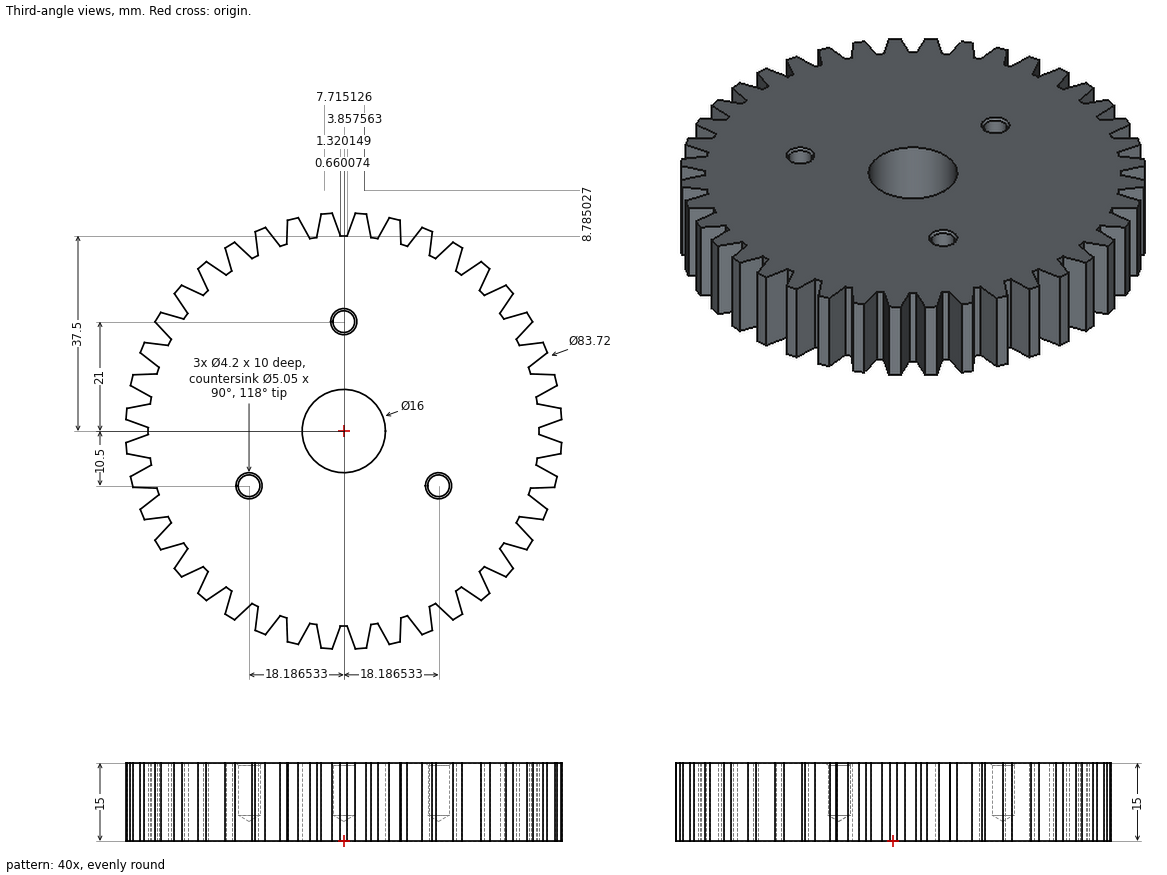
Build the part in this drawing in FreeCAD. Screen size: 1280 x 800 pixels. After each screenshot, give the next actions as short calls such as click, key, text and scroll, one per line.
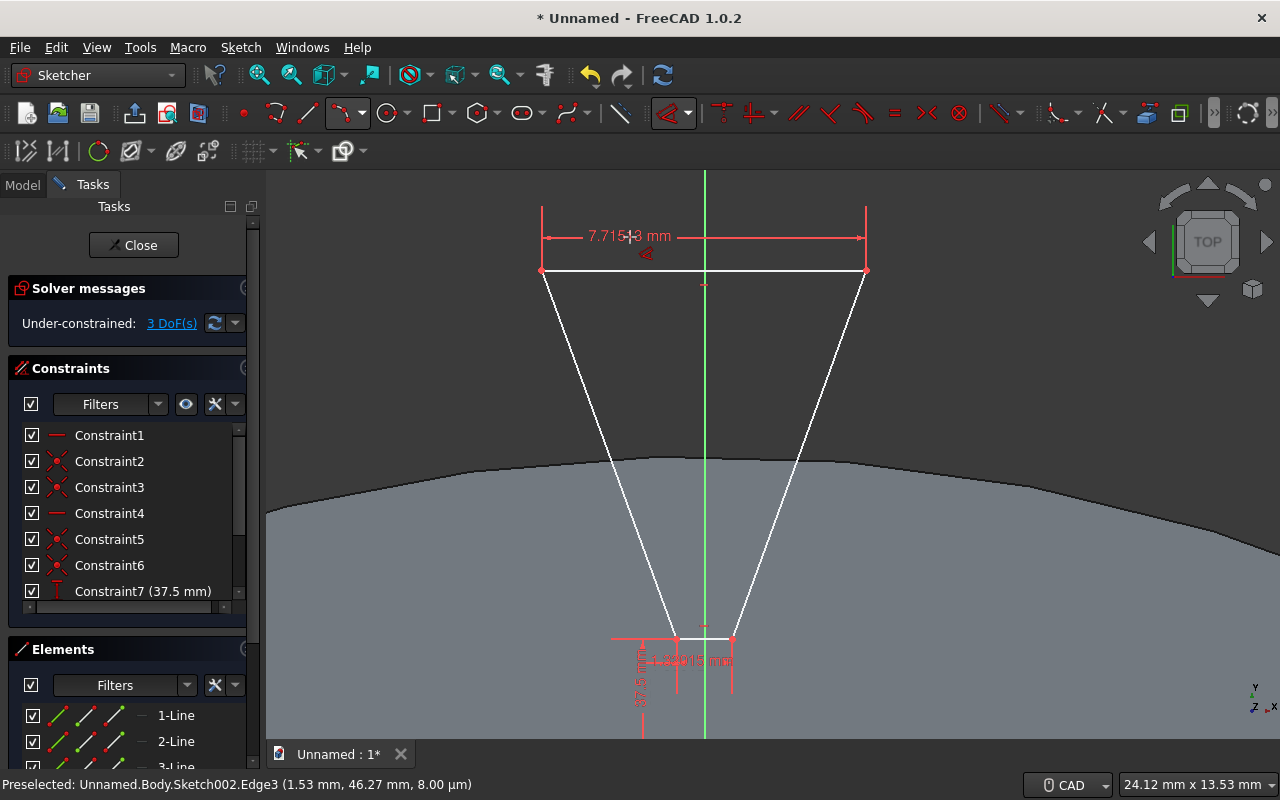
scroll(677, 639, up, 2)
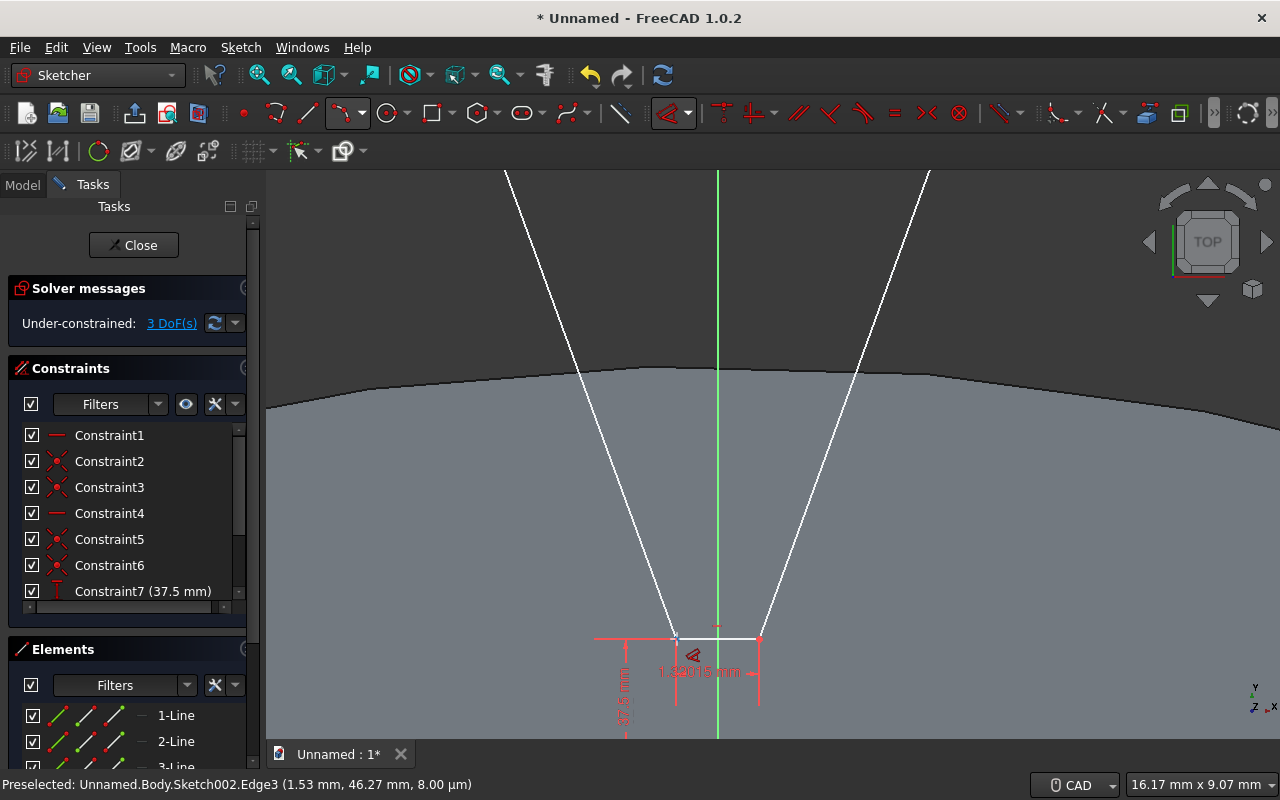
click(676, 639)
click(697, 605)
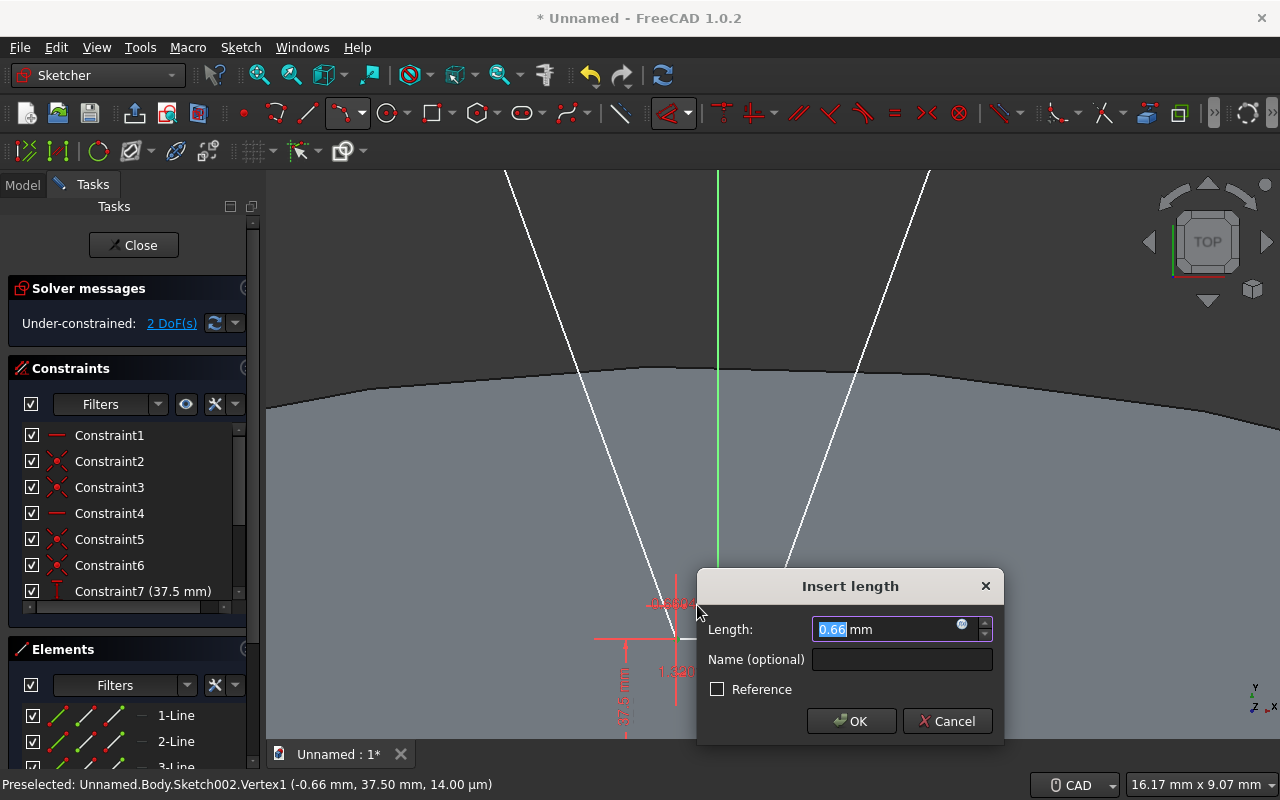
text(0.660074)
key(Return)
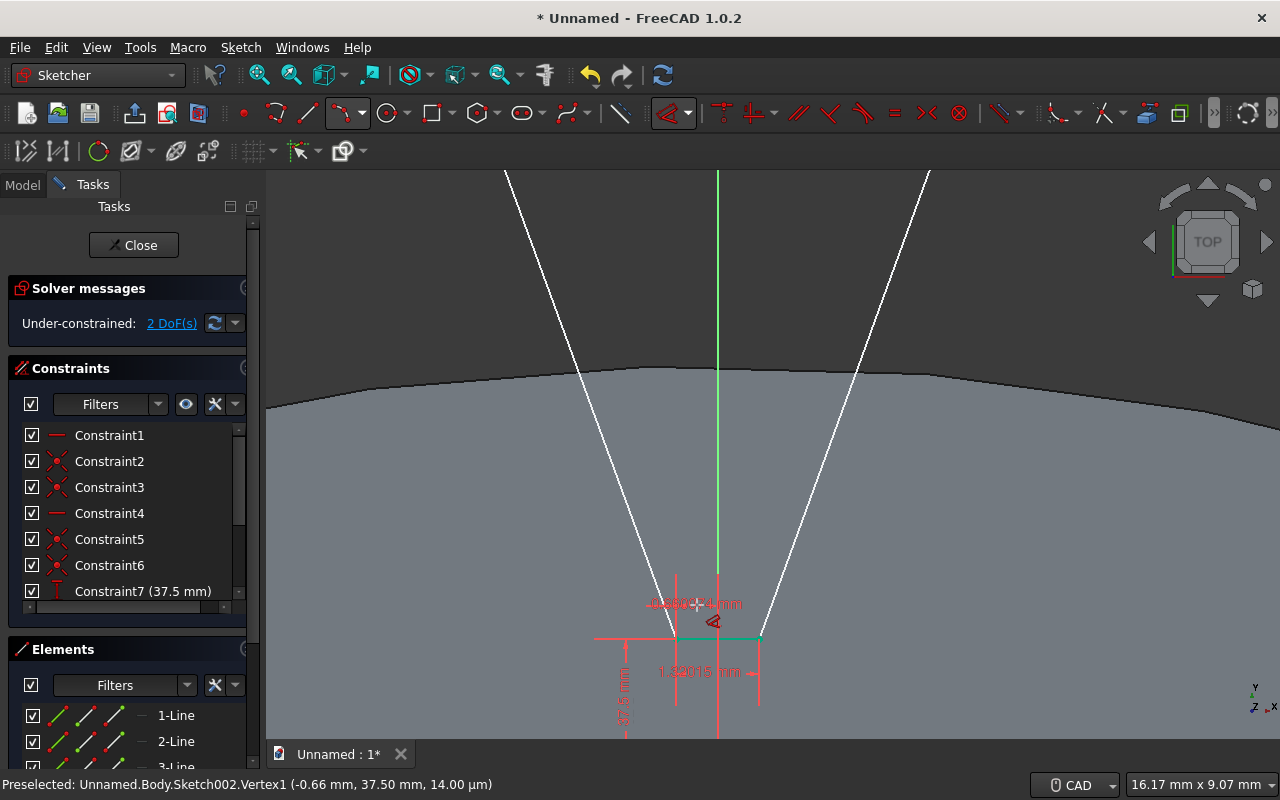
scroll(677, 639, down, 2)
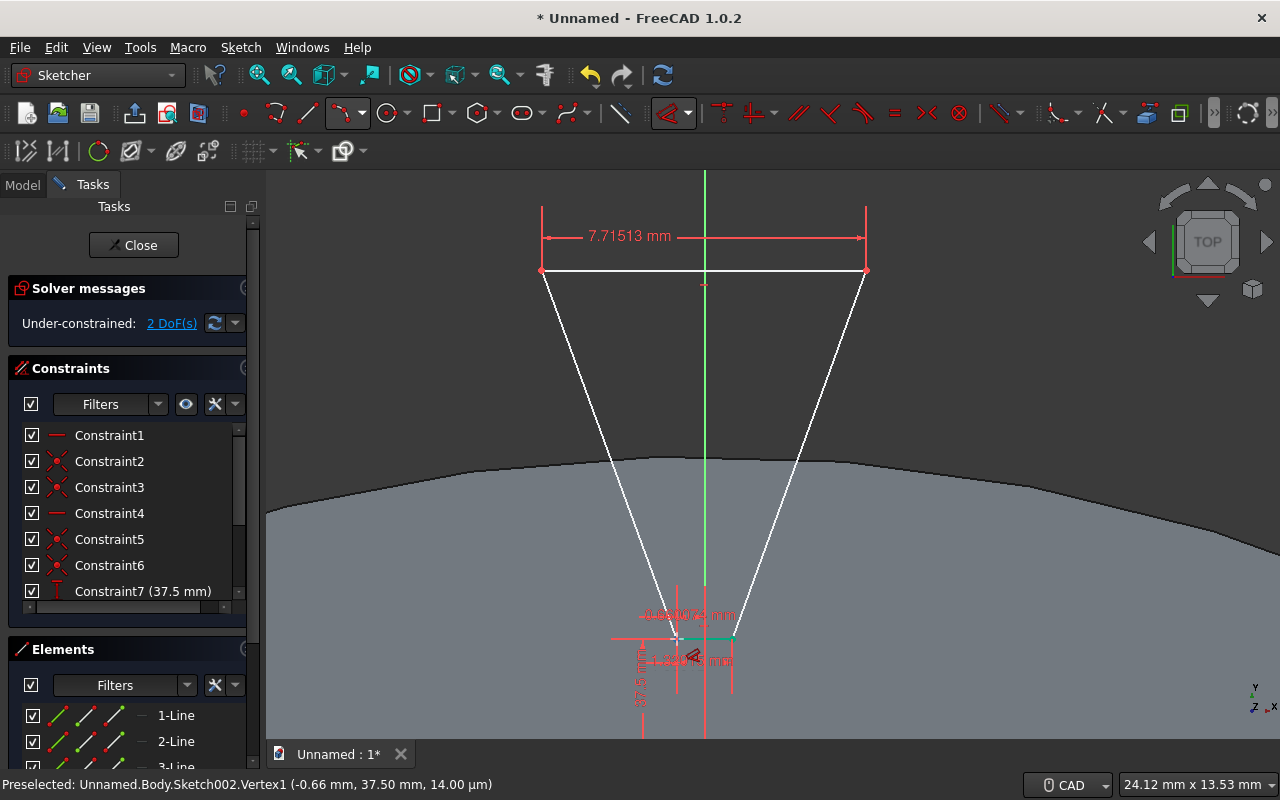
click(866, 271)
click(785, 237)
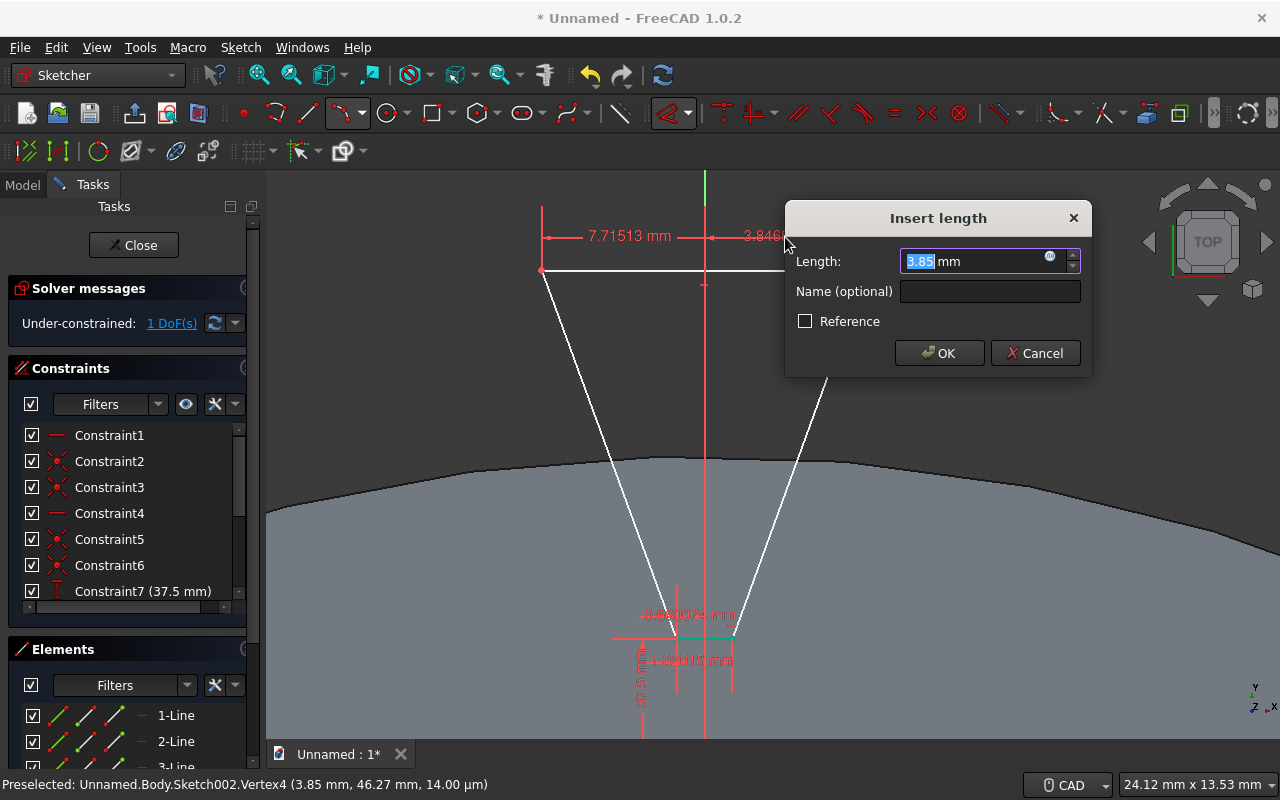
text(3.857563)
key(Return)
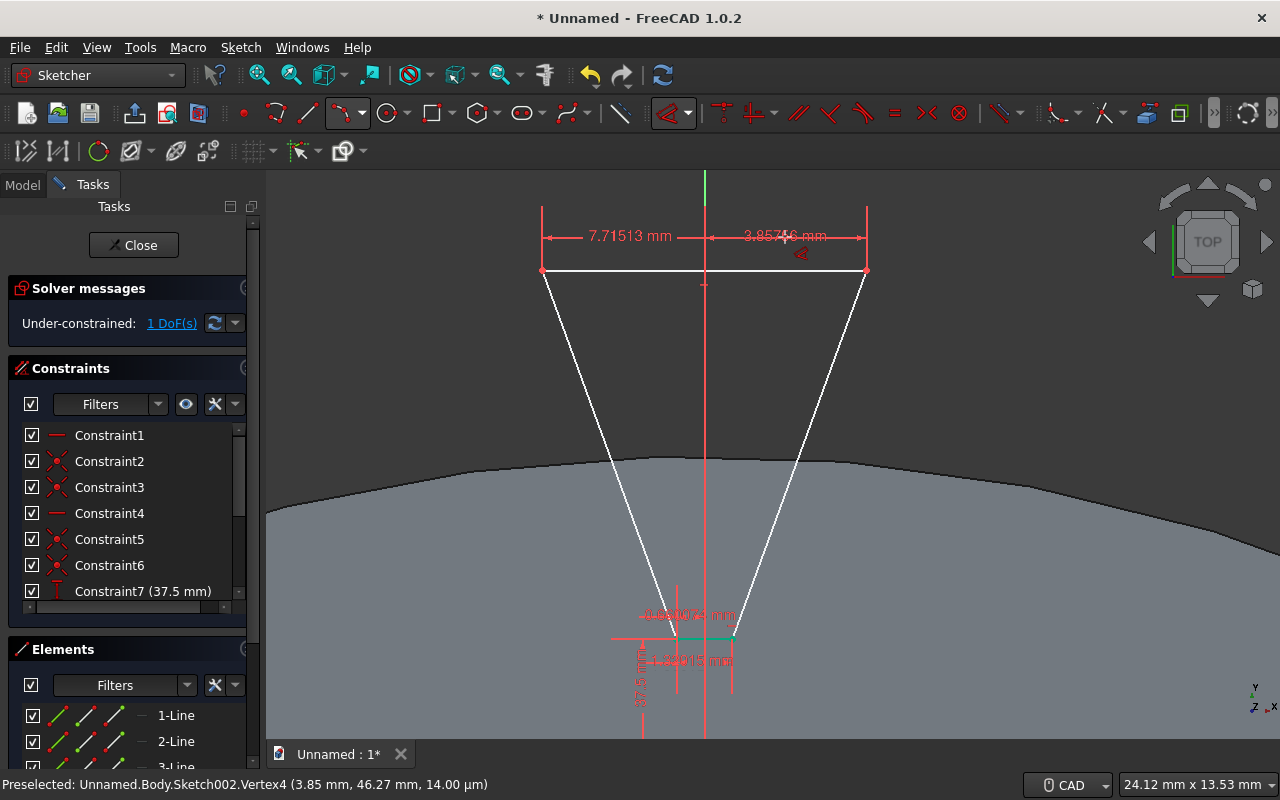
click(773, 529)
click(901, 455)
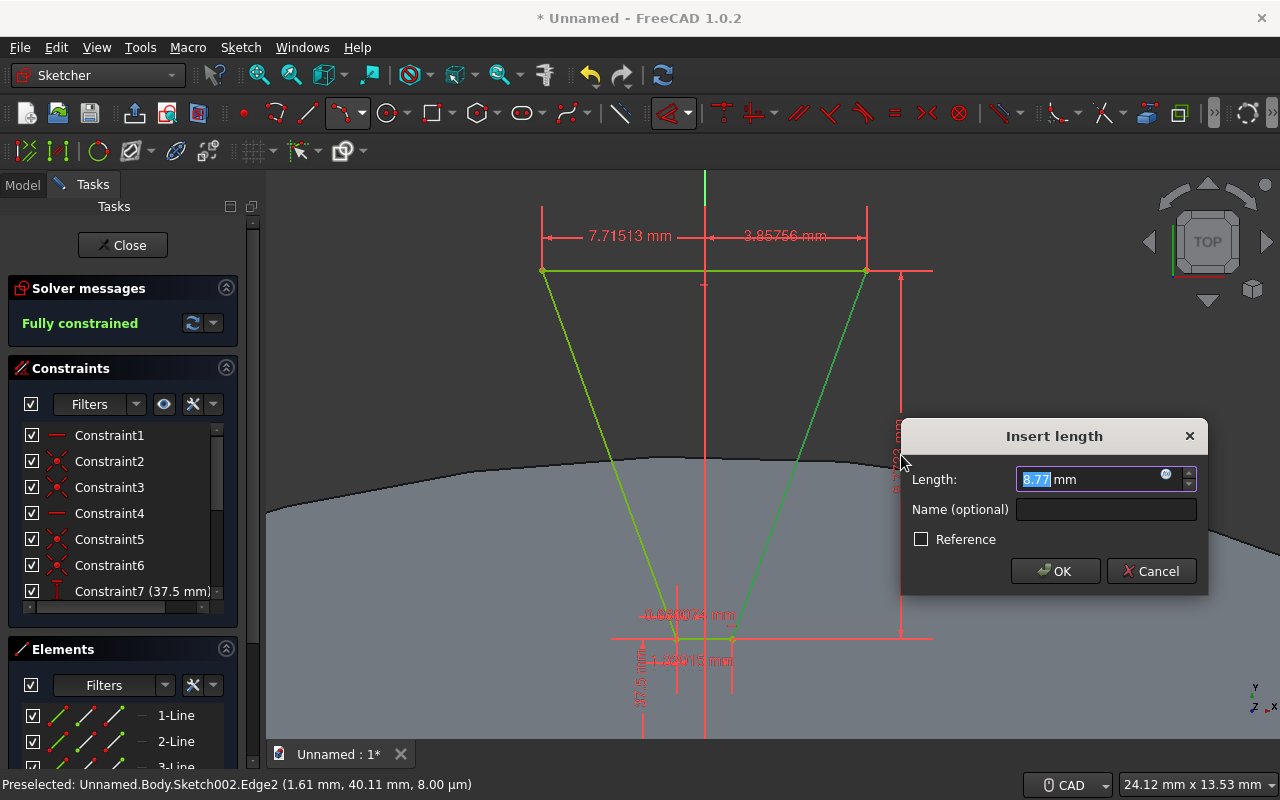
text(8.785027)
key(Return)
key(Escape)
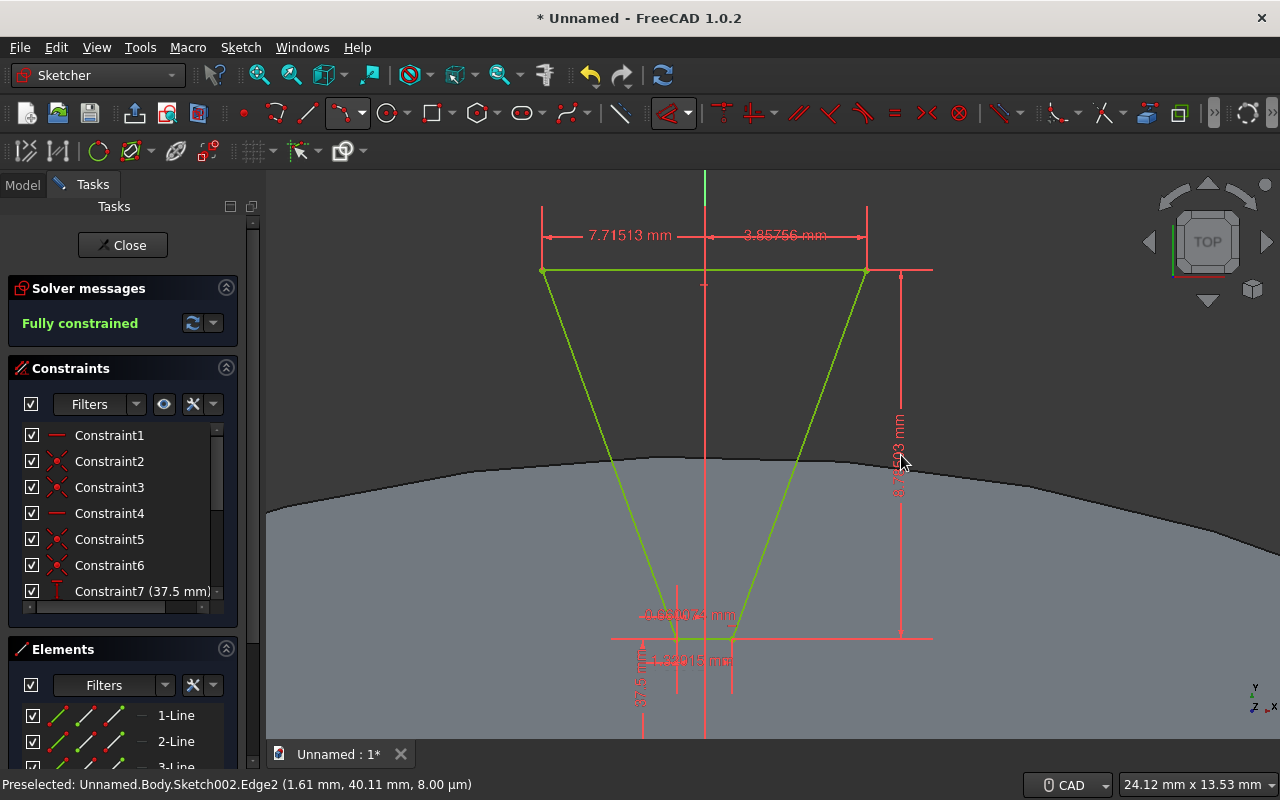
click(123, 245)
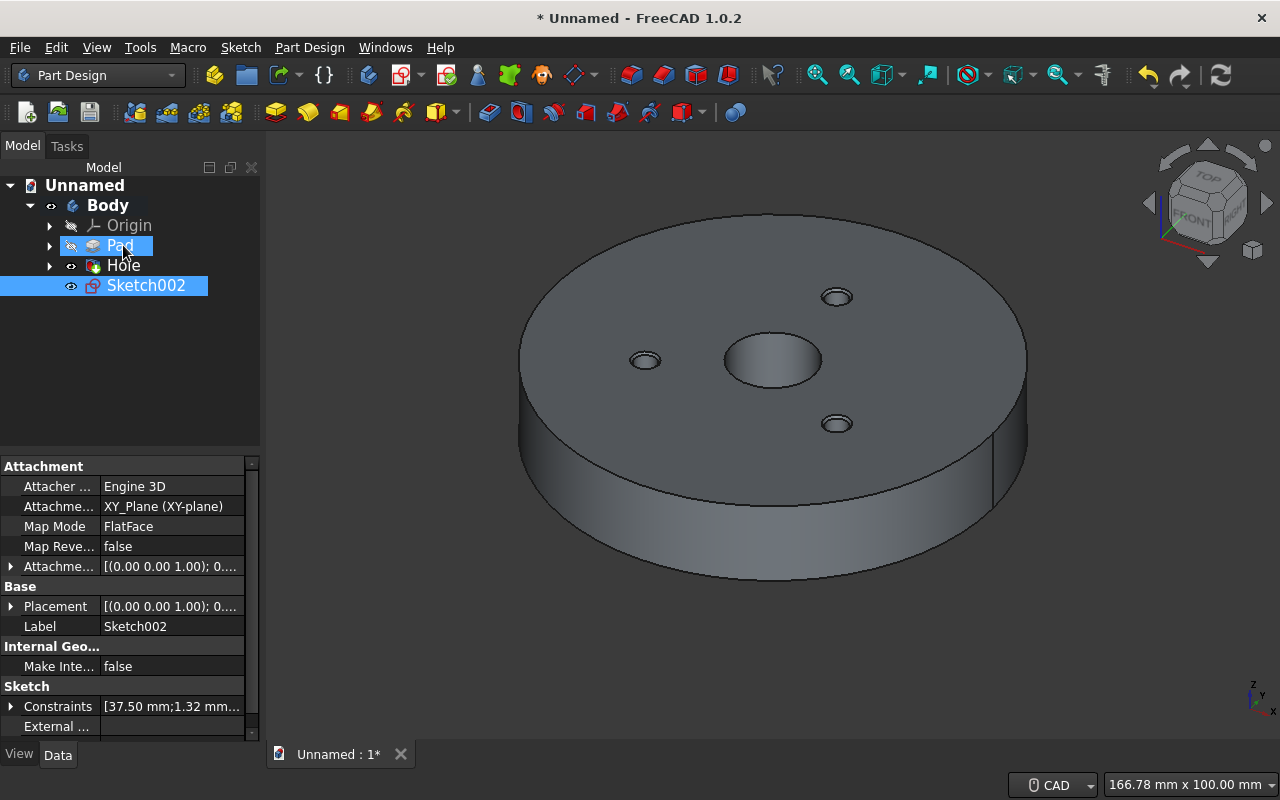
click(490, 112)